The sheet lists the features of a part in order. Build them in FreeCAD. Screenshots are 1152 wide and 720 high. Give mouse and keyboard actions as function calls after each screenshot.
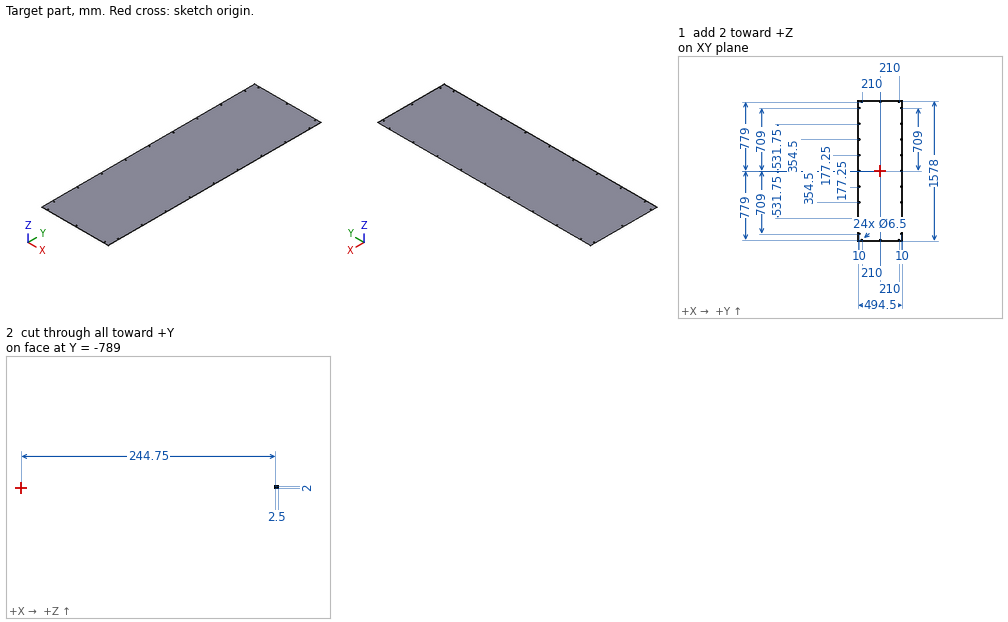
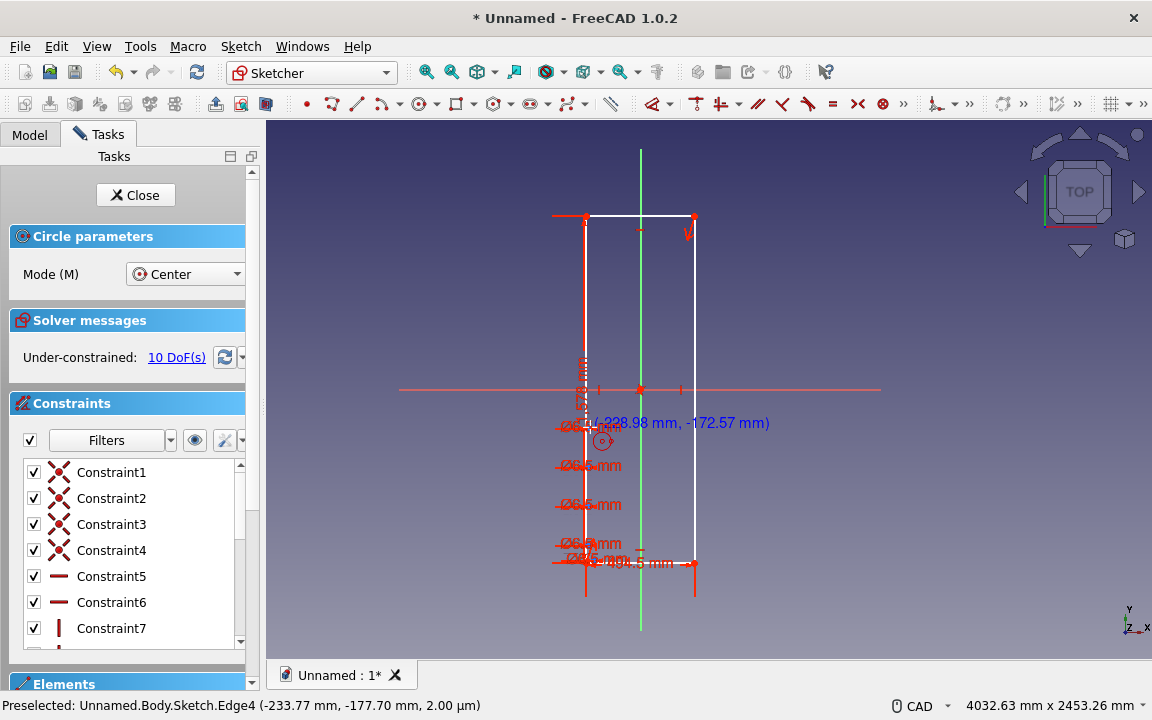
scroll(641, 561, up, 18)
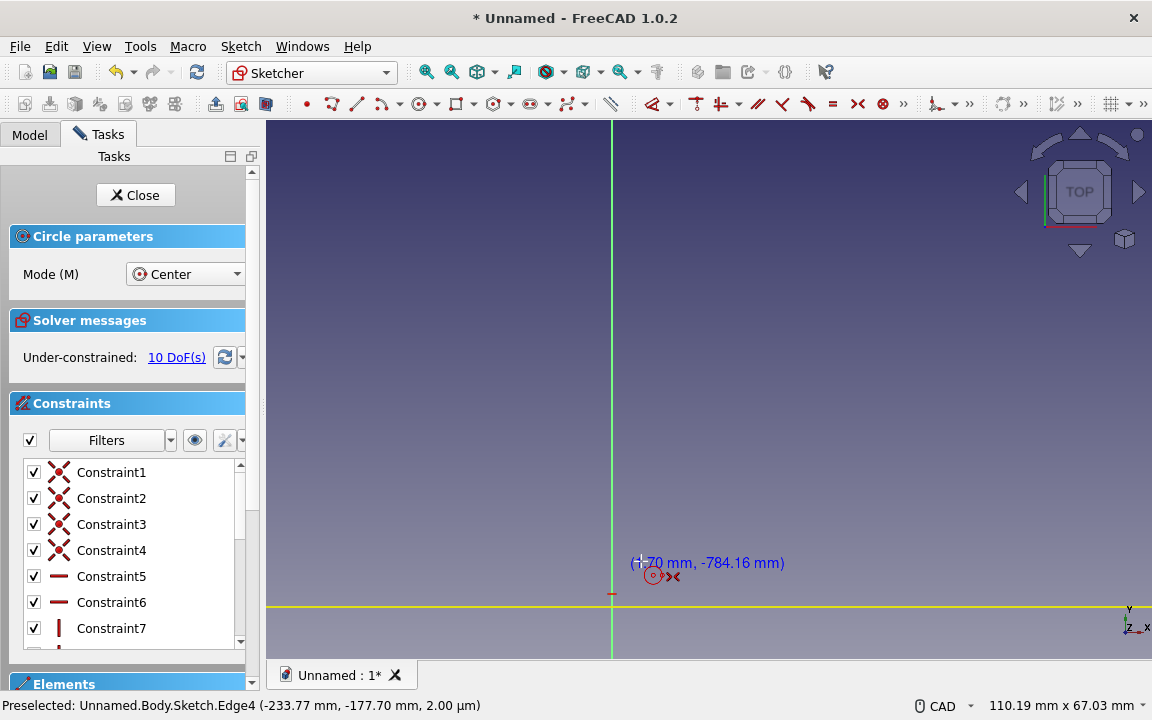
scroll(641, 601, down, 17)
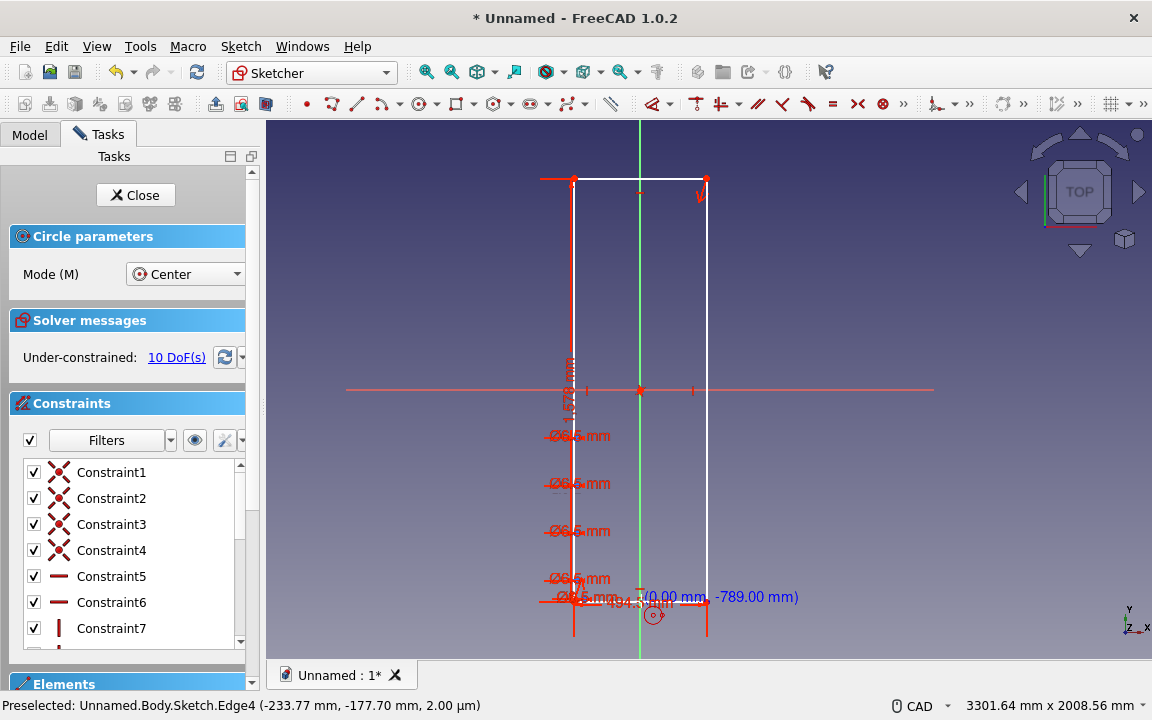
scroll(640, 599, up, 9)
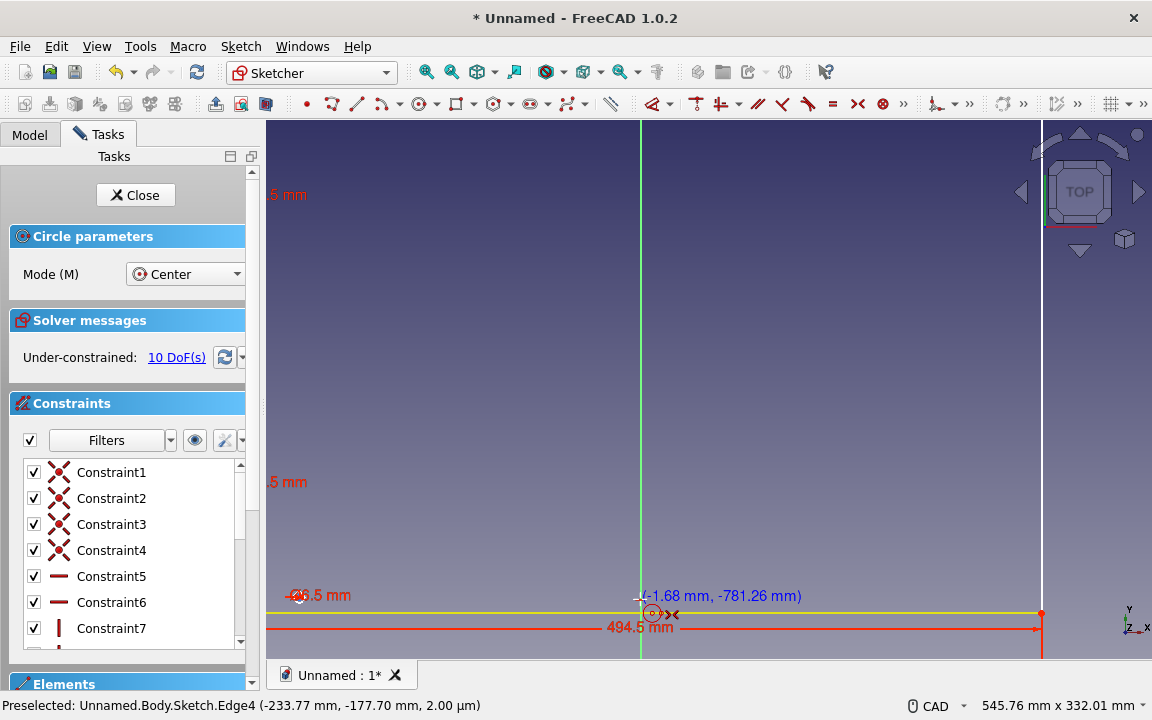
click(641, 597)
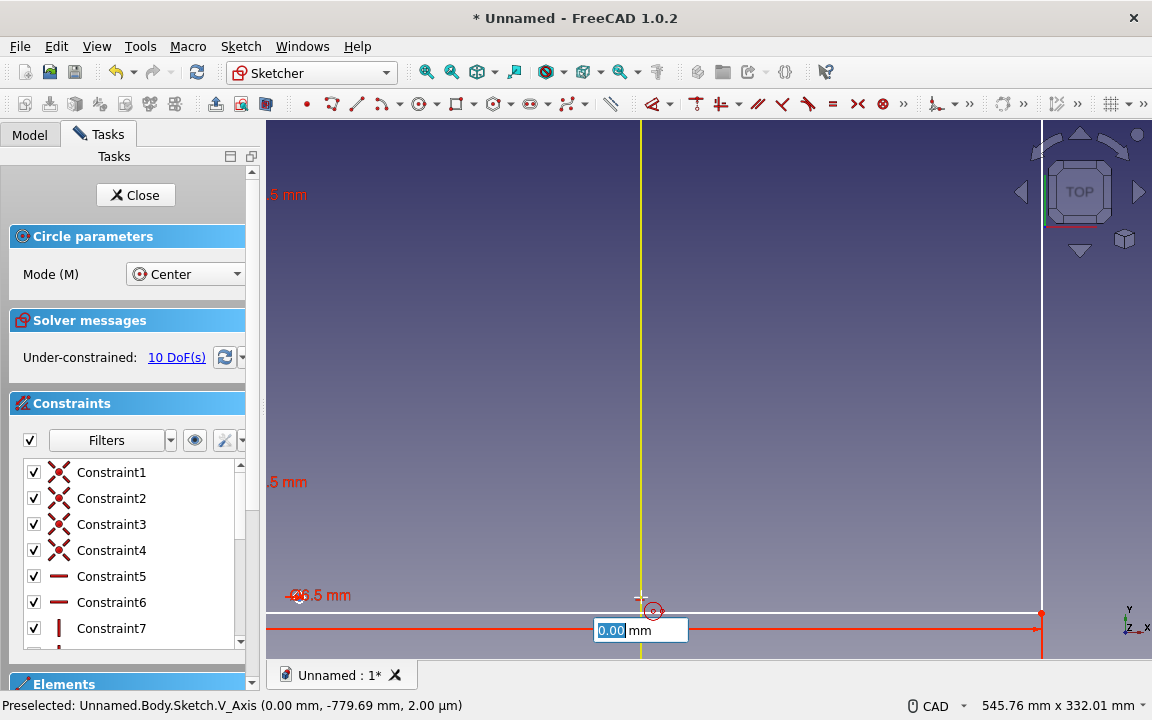
scroll(646, 595, up, 6)
move(643, 593)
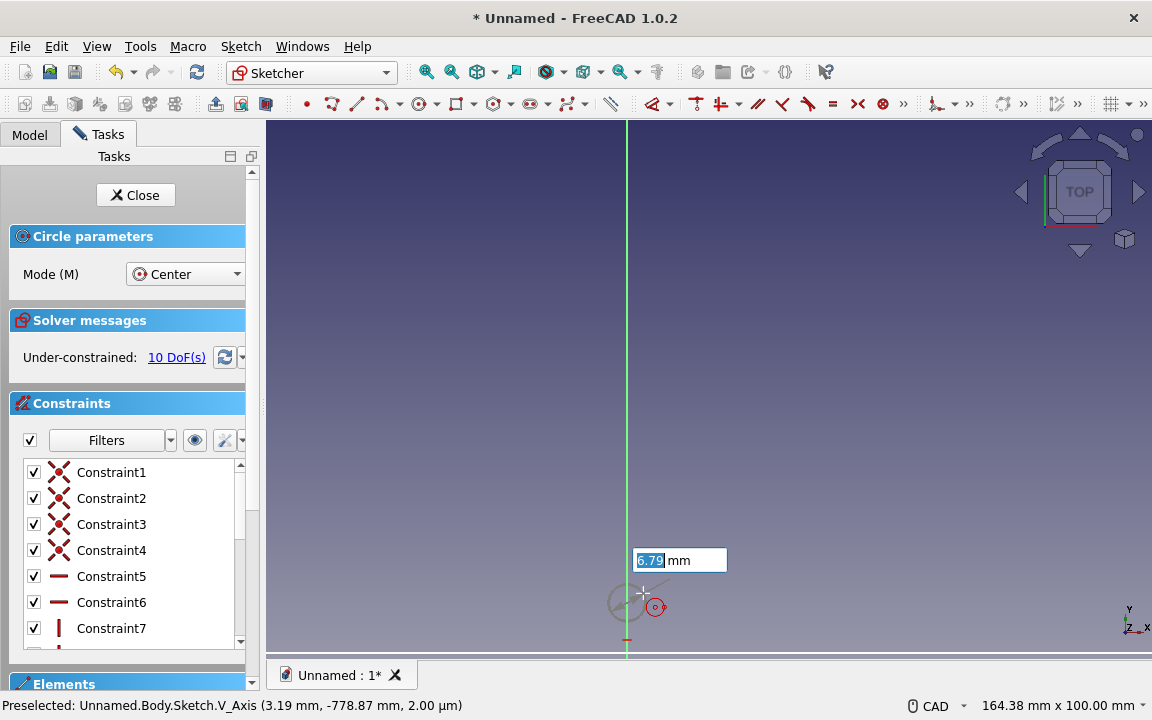
text(6.5)
key(Return)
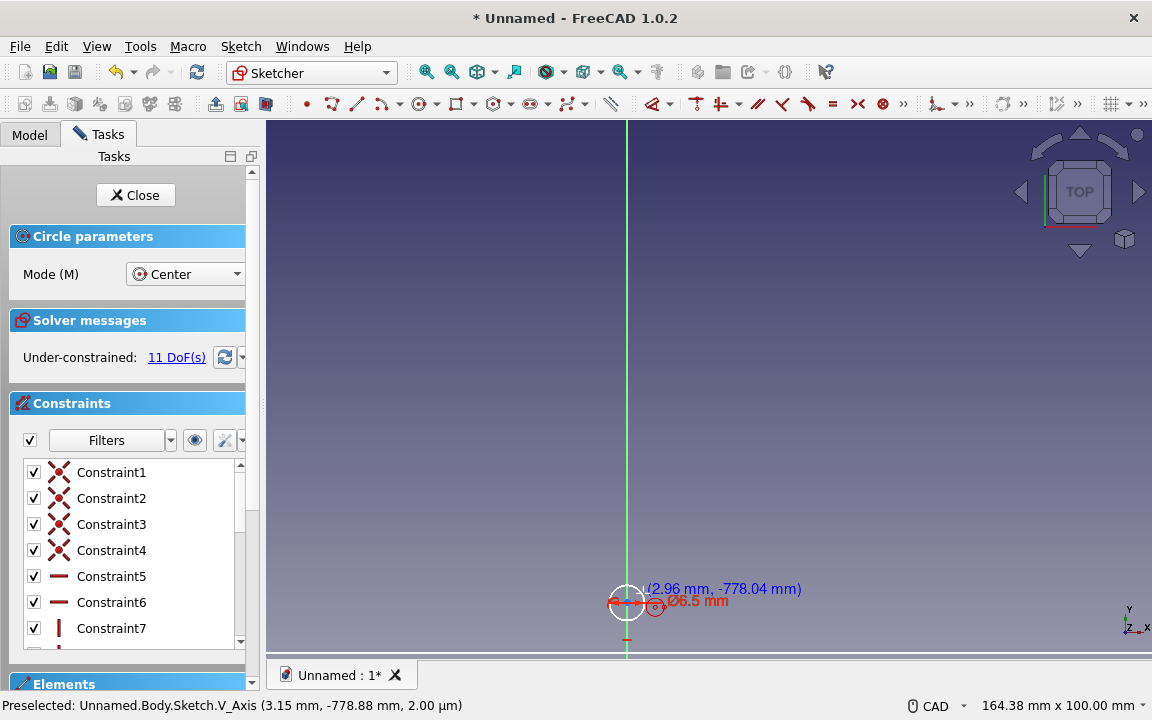
scroll(641, 599, down, 15)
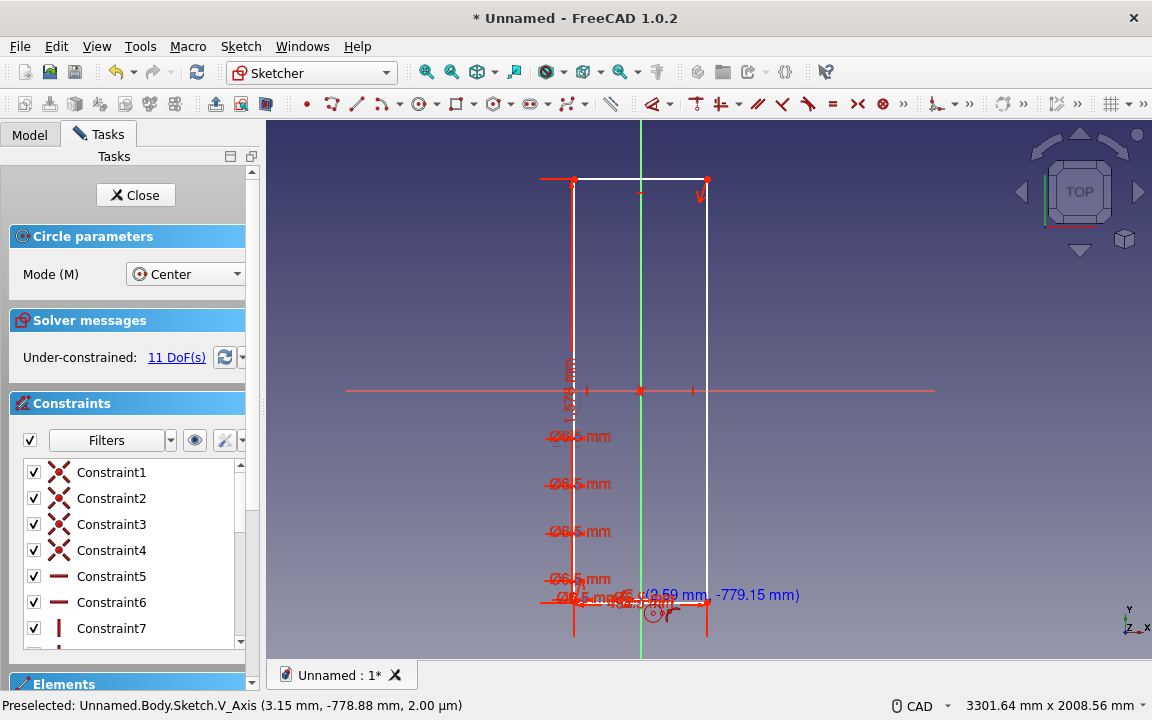
scroll(697, 600, up, 17)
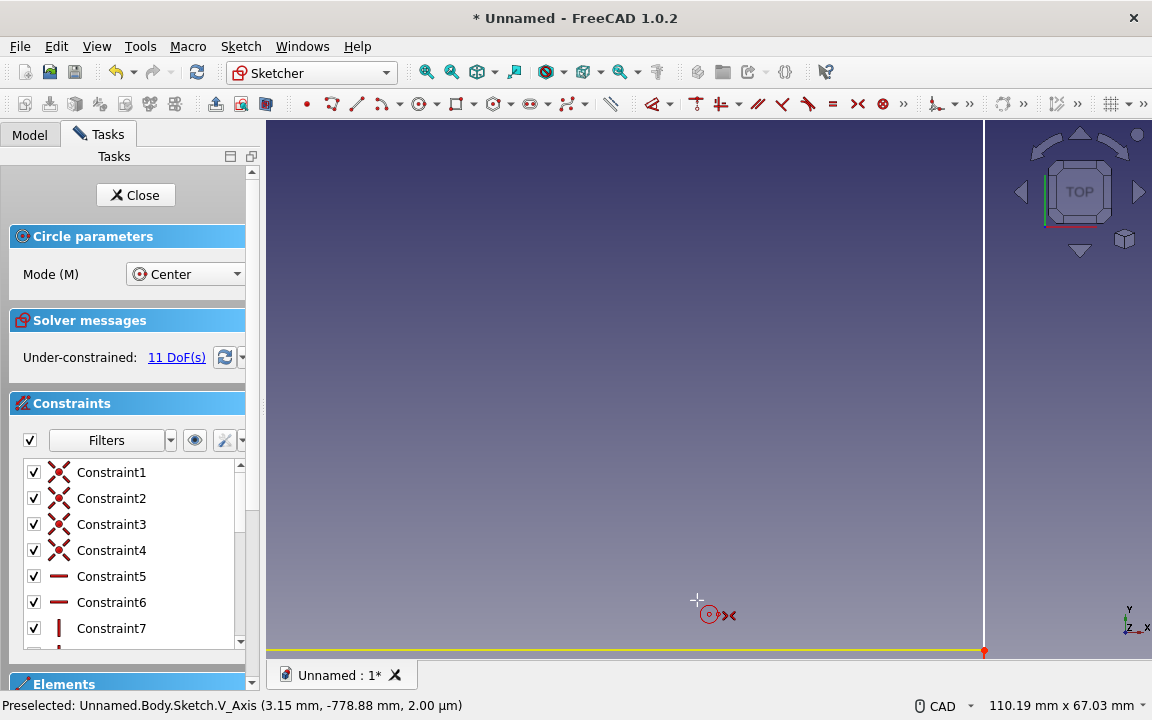
scroll(697, 600, down, 17)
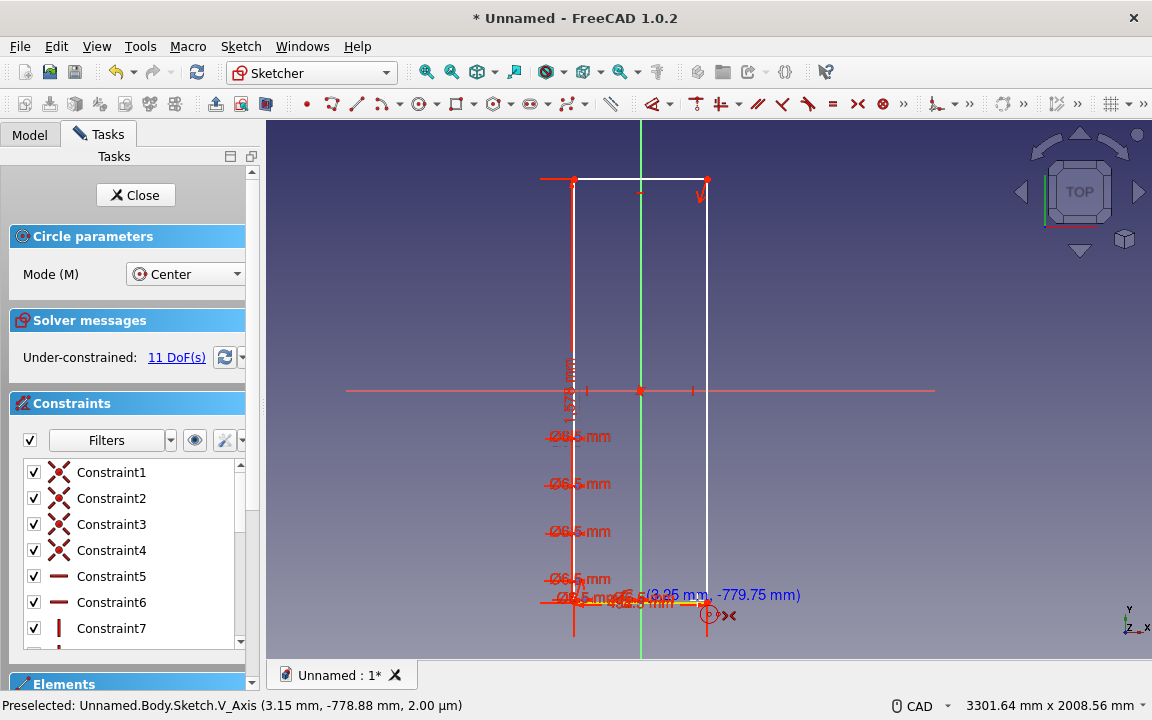
scroll(697, 600, up, 9)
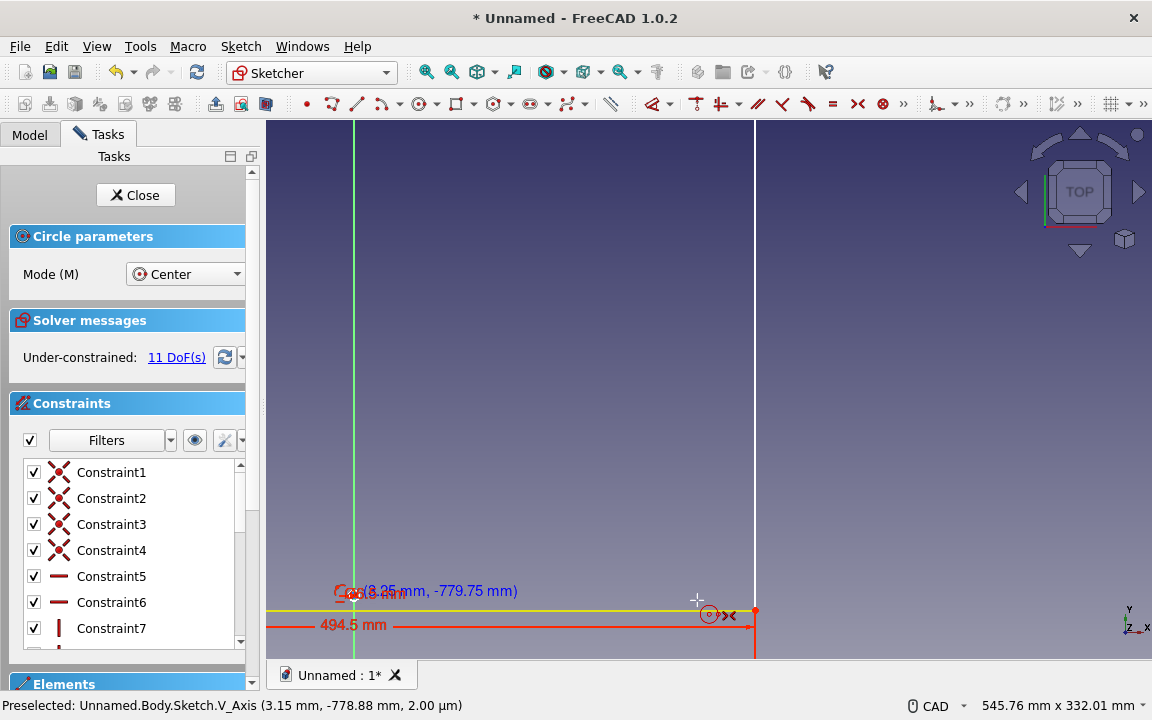
click(695, 595)
move(699, 591)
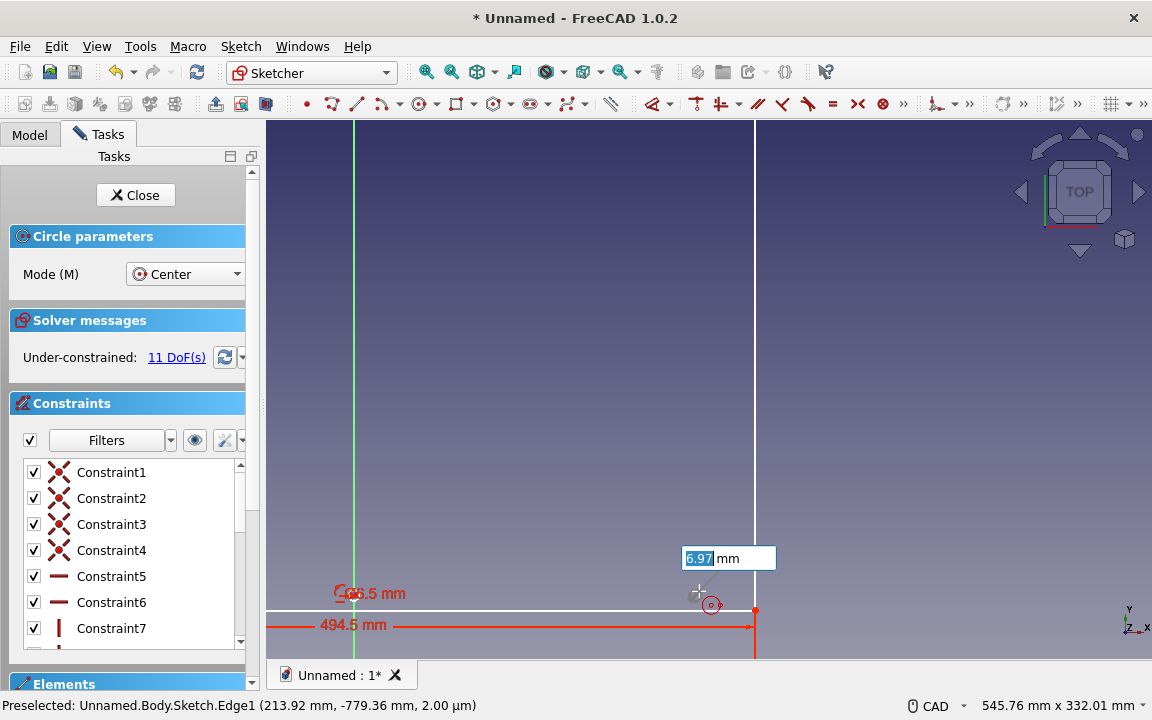
text(6.5)
key(Return)